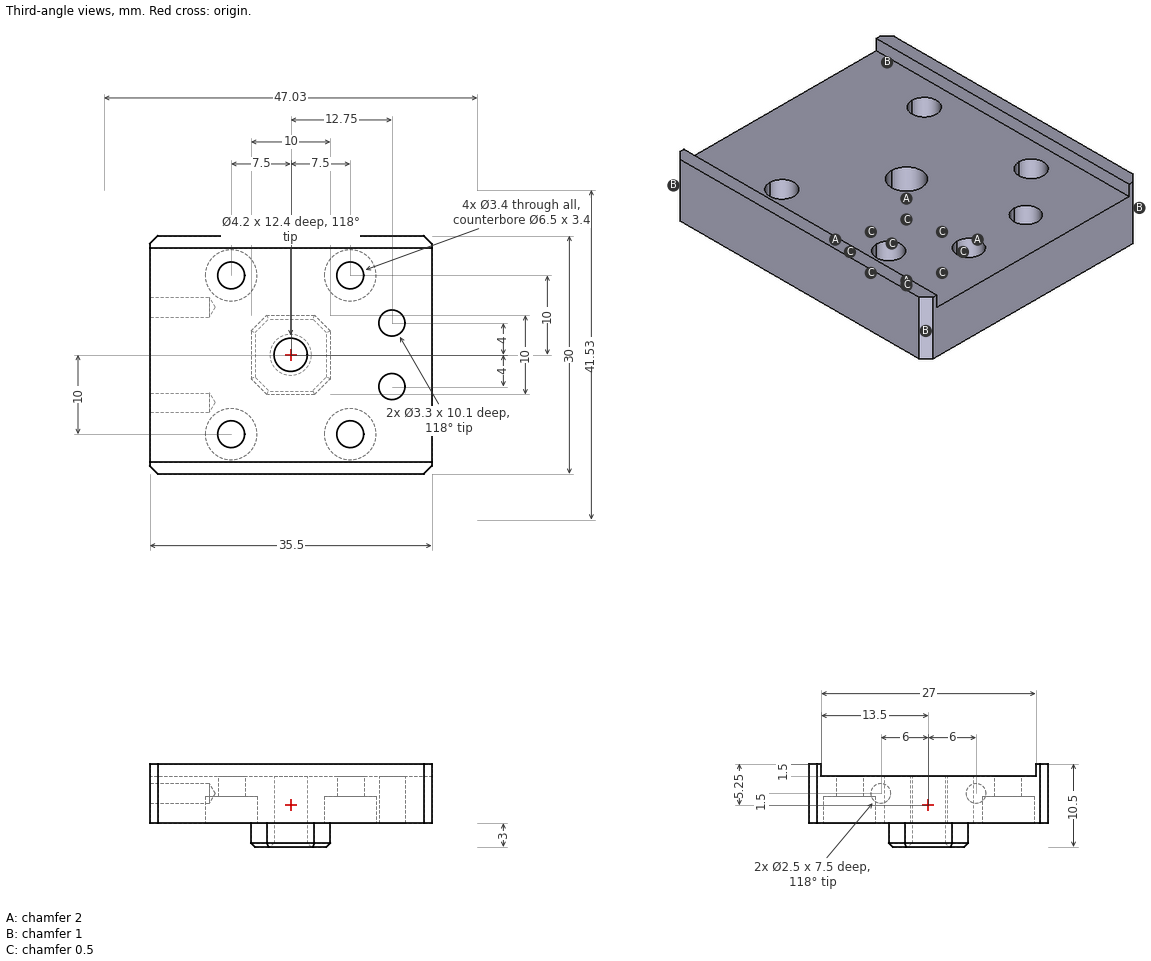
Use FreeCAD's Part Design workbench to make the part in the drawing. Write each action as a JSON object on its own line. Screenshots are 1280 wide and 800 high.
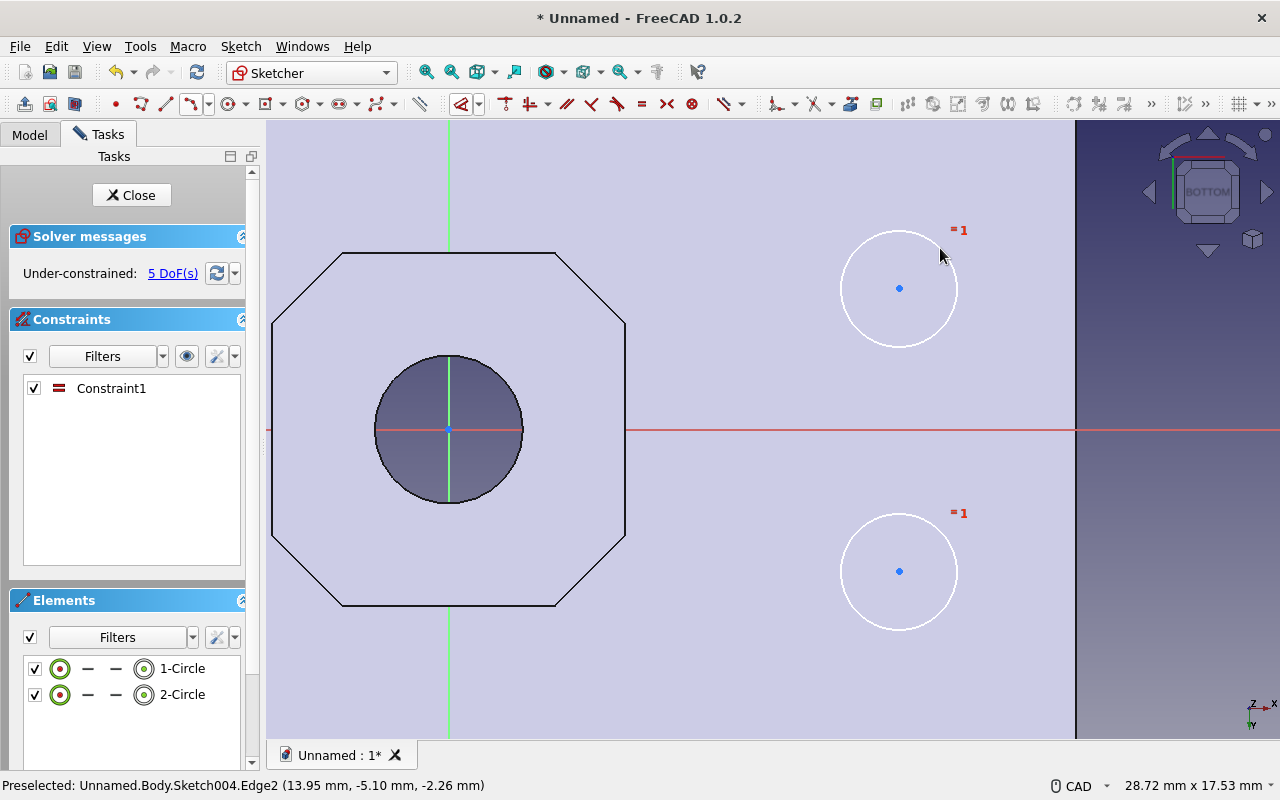
{"action": "left_click", "coordinate": [899, 572]}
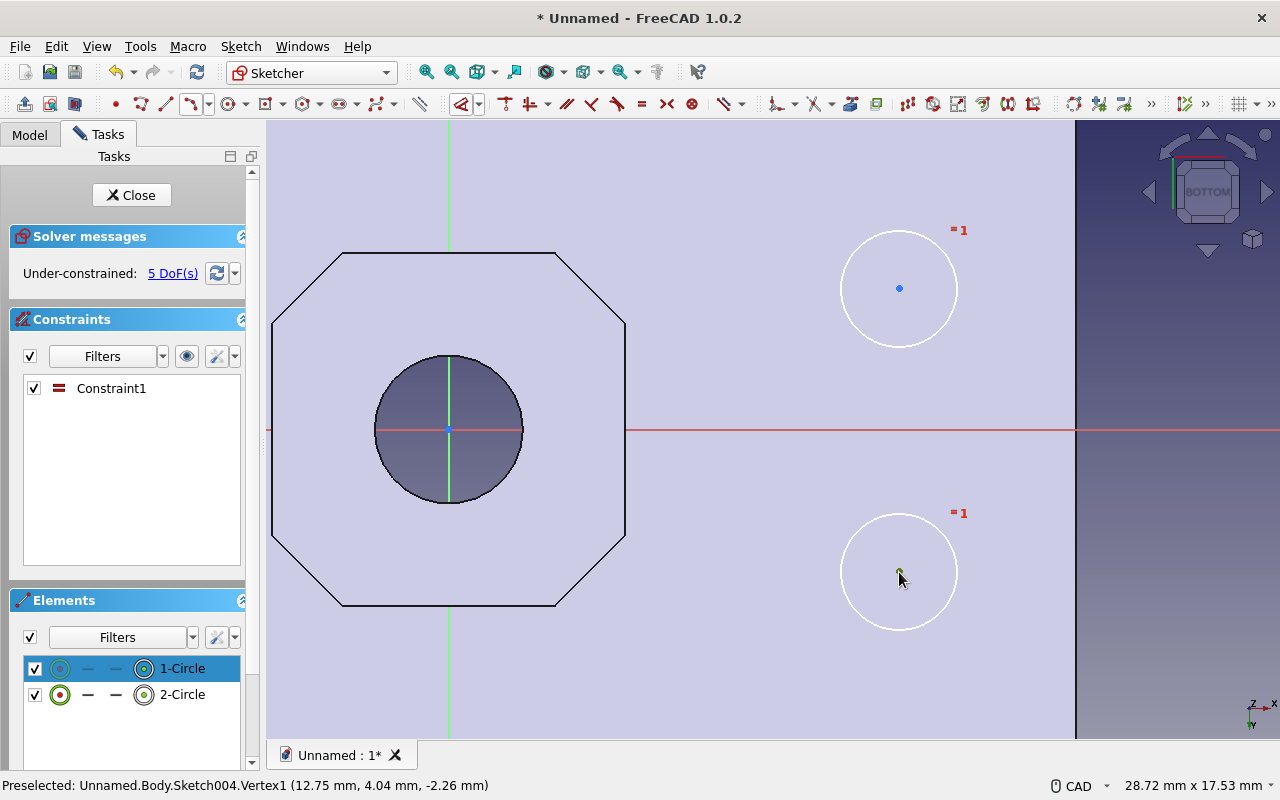
{"action": "left_click", "coordinate": [899, 289]}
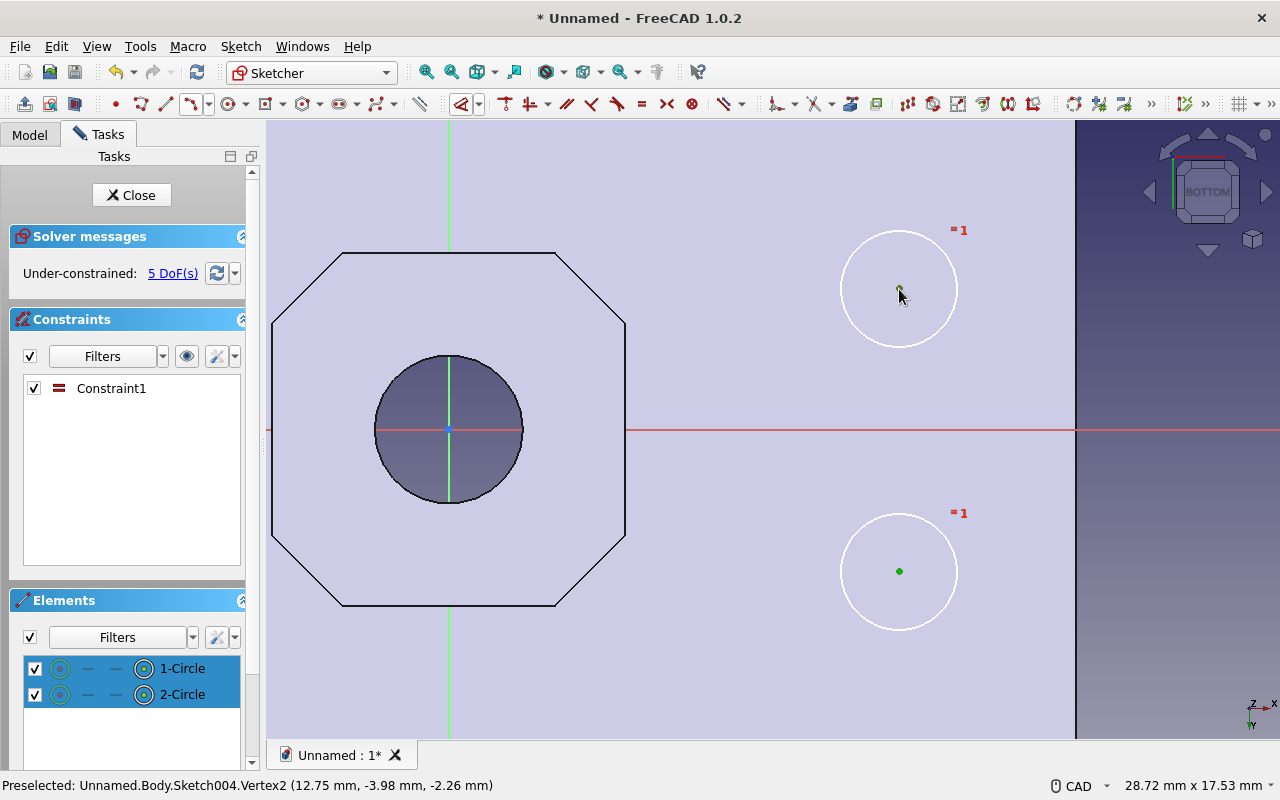
{"action": "key", "text": "v"}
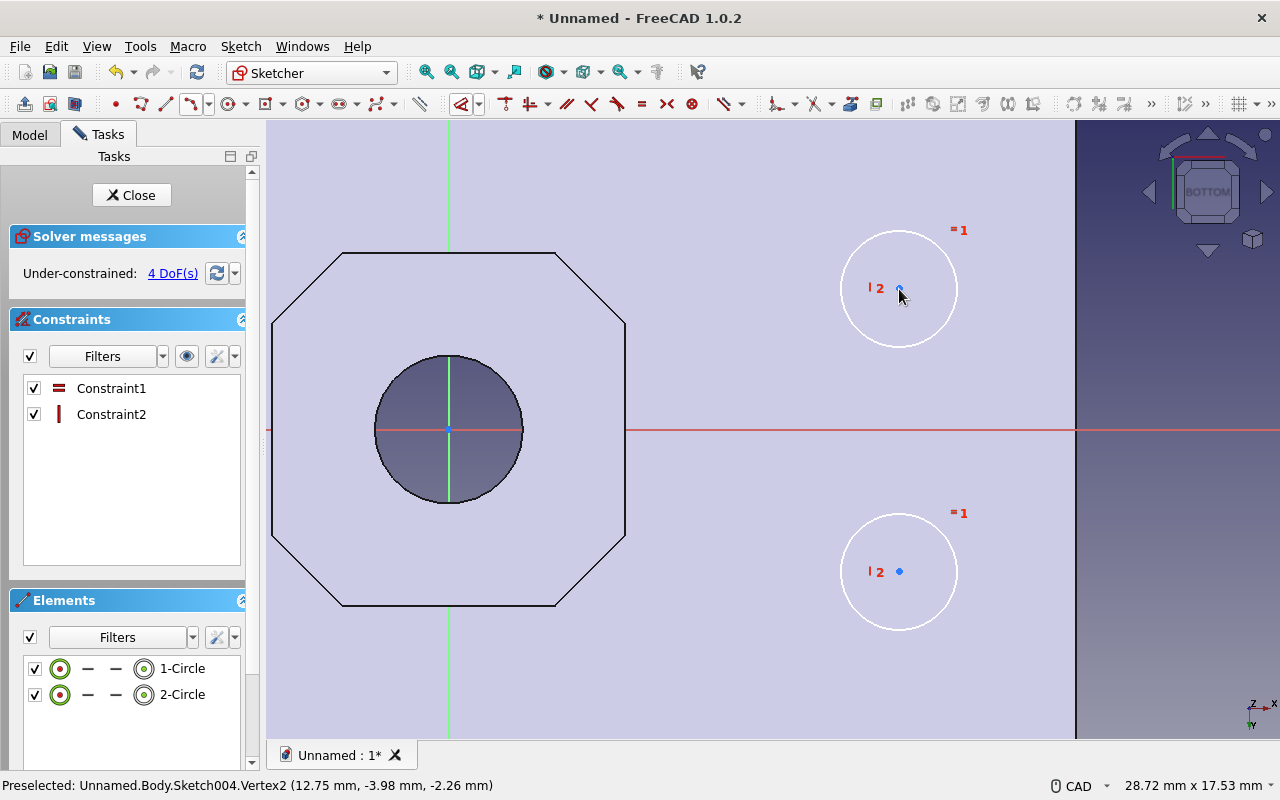
{"action": "key", "text": "d"}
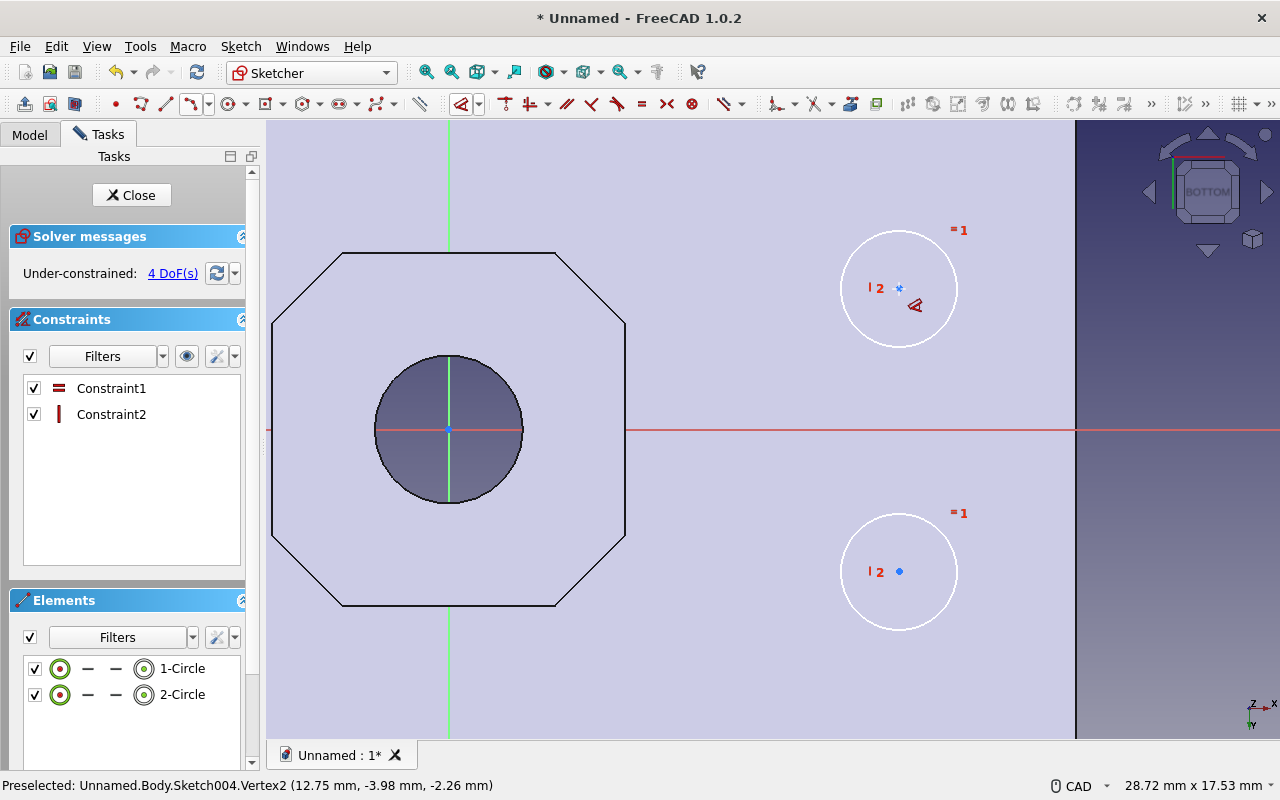
{"action": "left_click", "coordinate": [940, 531]}
{"action": "left_click", "coordinate": [963, 508]}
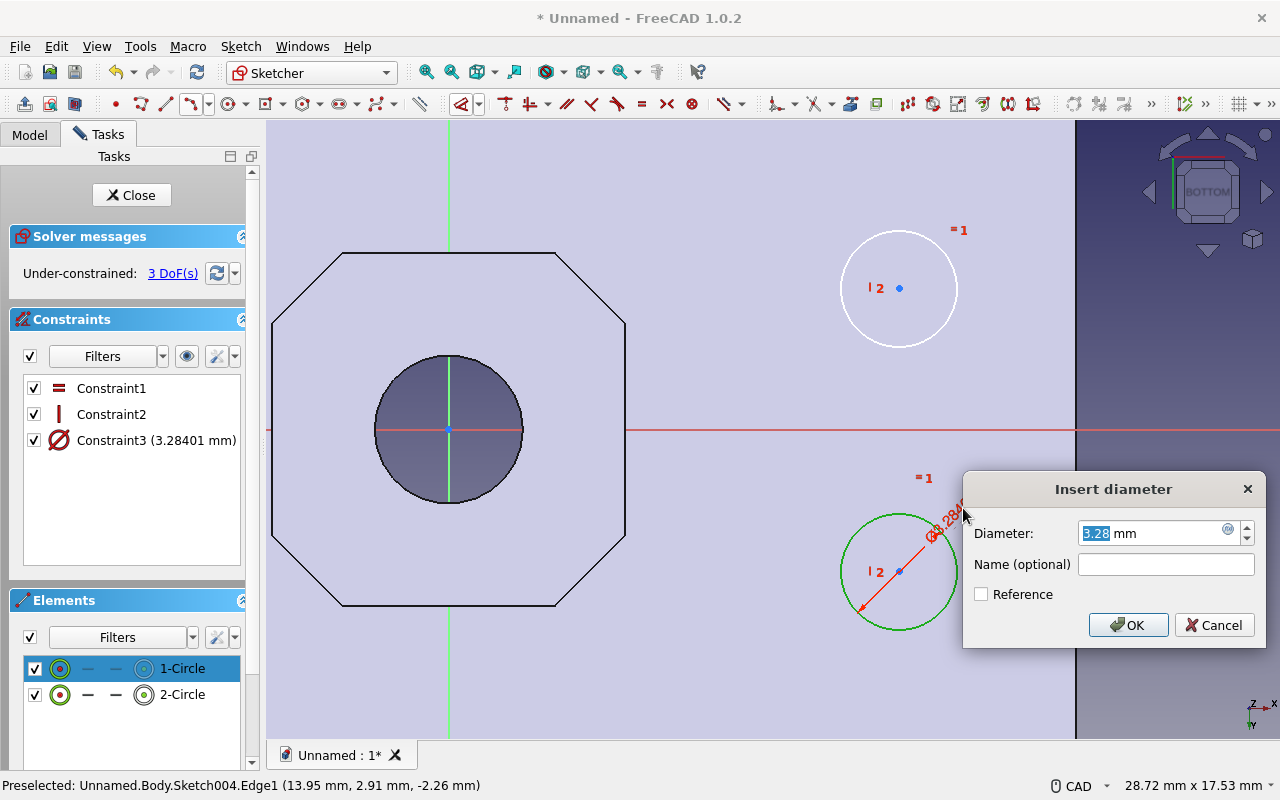
{"action": "type", "text": "3.3"}
{"action": "key", "text": "Return"}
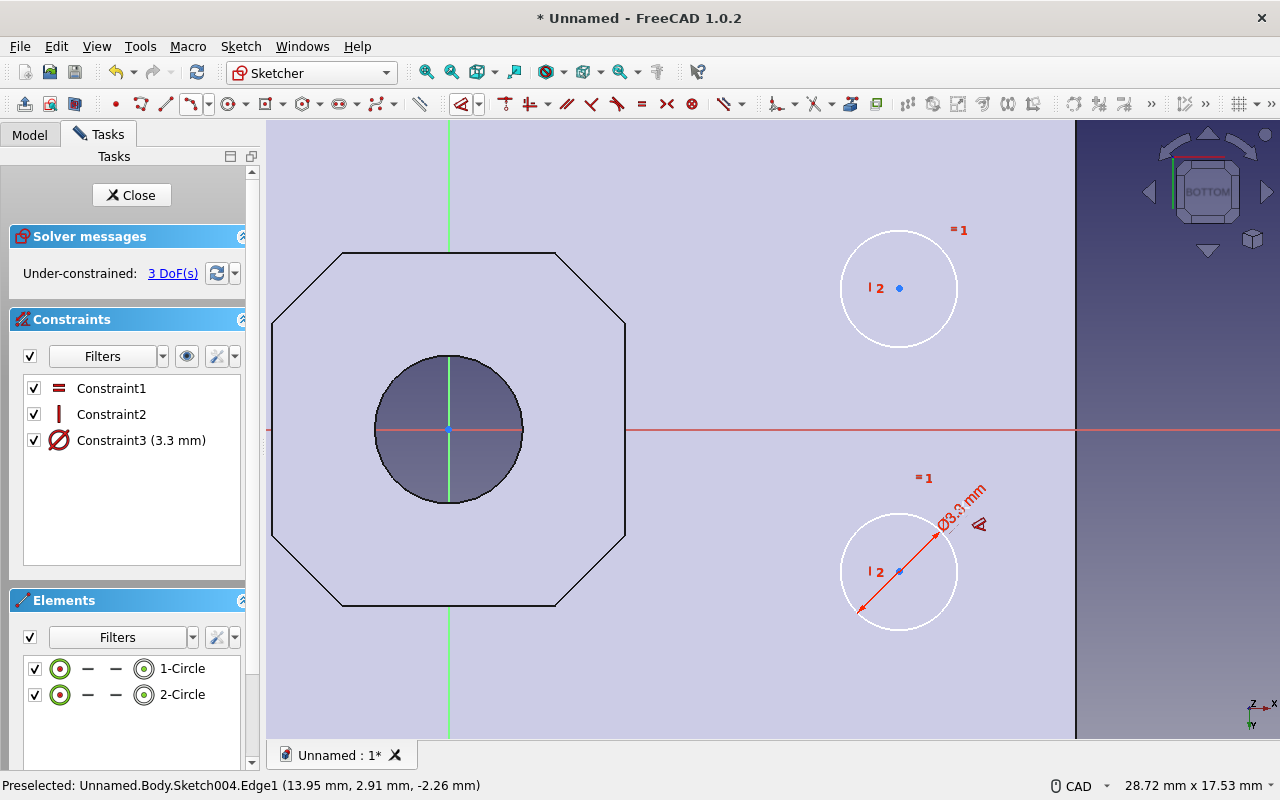
{"action": "left_click", "coordinate": [899, 572]}
{"action": "left_click", "coordinate": [415, 501]}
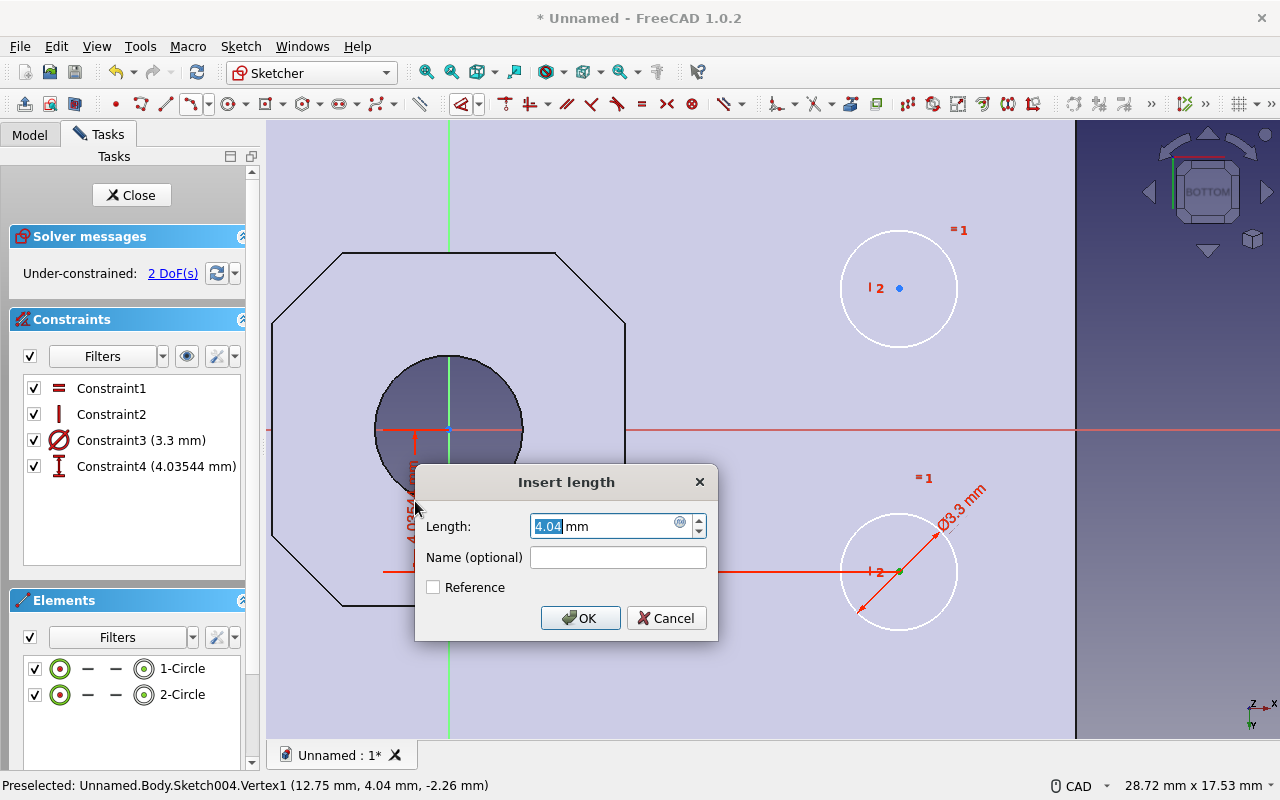
{"action": "type", "text": "4"}
{"action": "key", "text": "Return"}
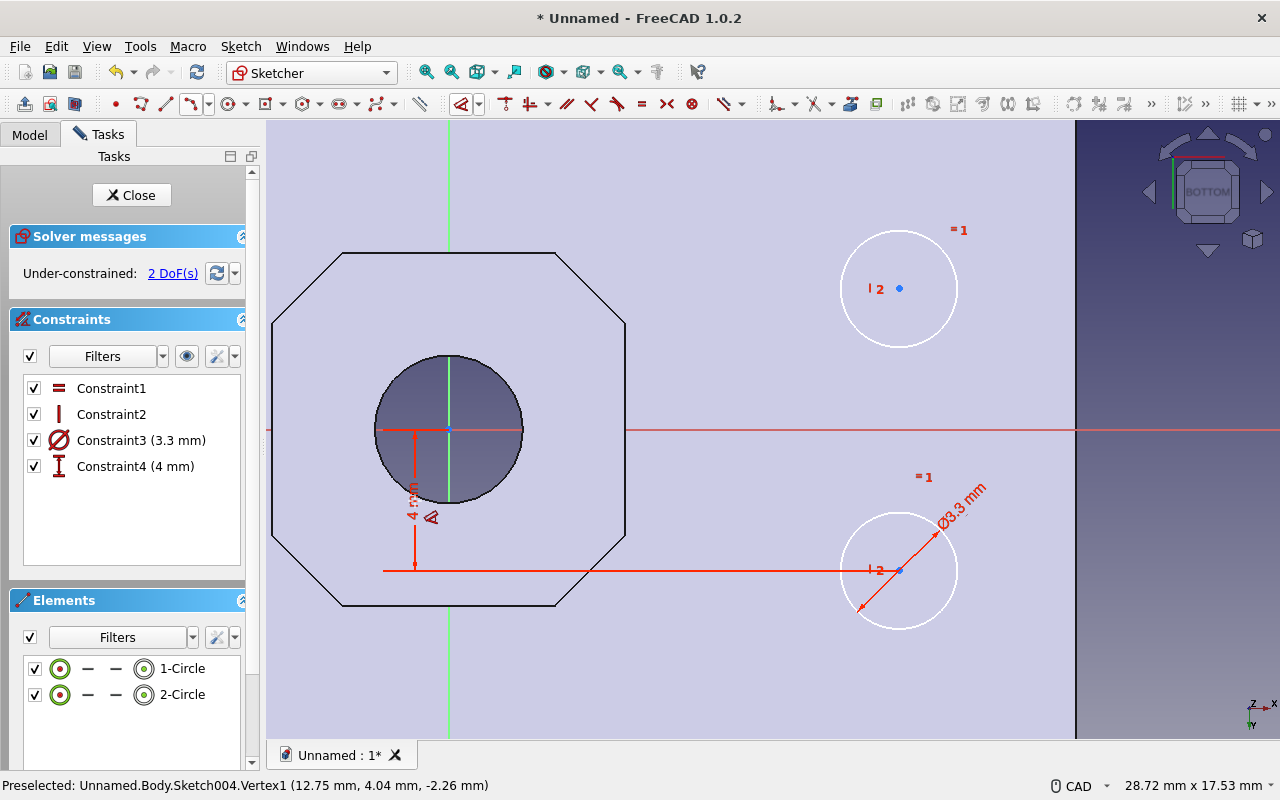
{"action": "left_click", "coordinate": [899, 289]}
{"action": "left_click", "coordinate": [415, 359]}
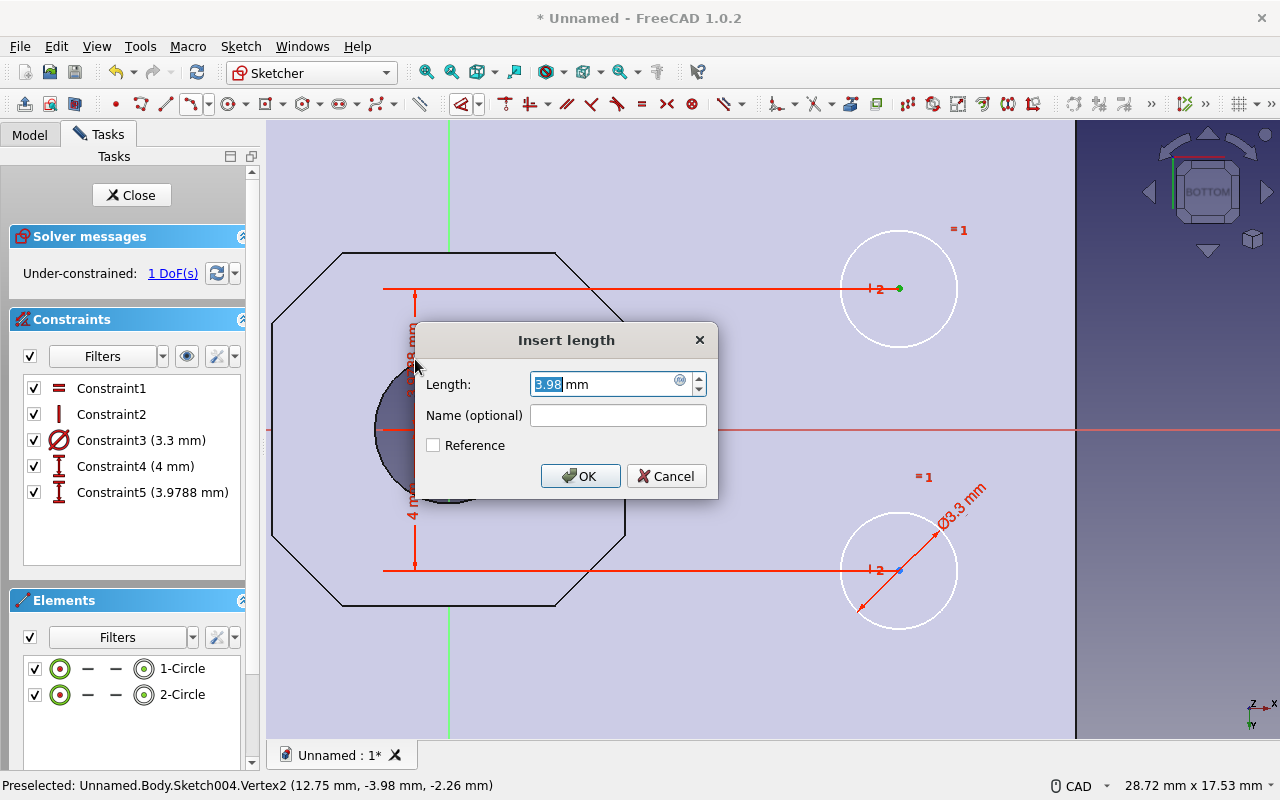
{"action": "type", "text": "4"}
{"action": "key", "text": "Return"}